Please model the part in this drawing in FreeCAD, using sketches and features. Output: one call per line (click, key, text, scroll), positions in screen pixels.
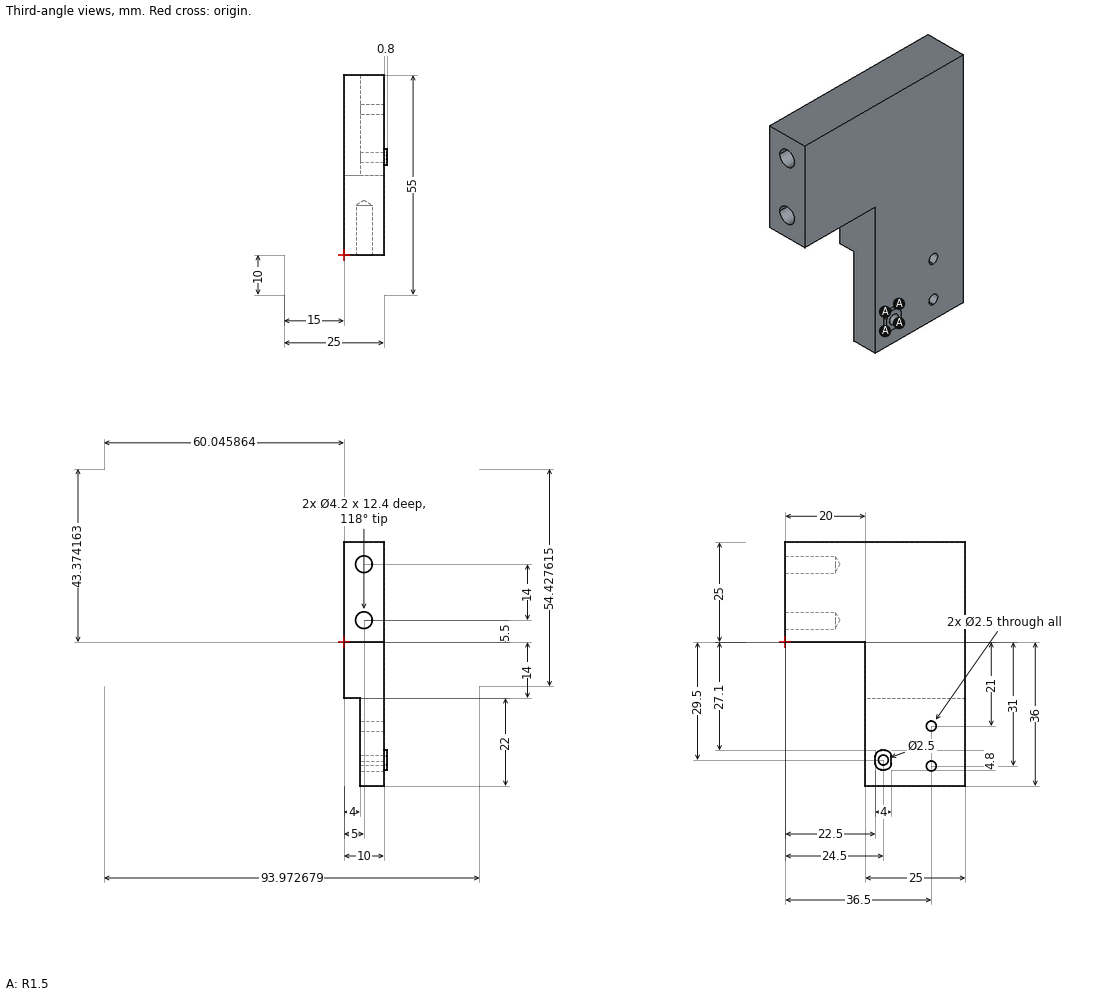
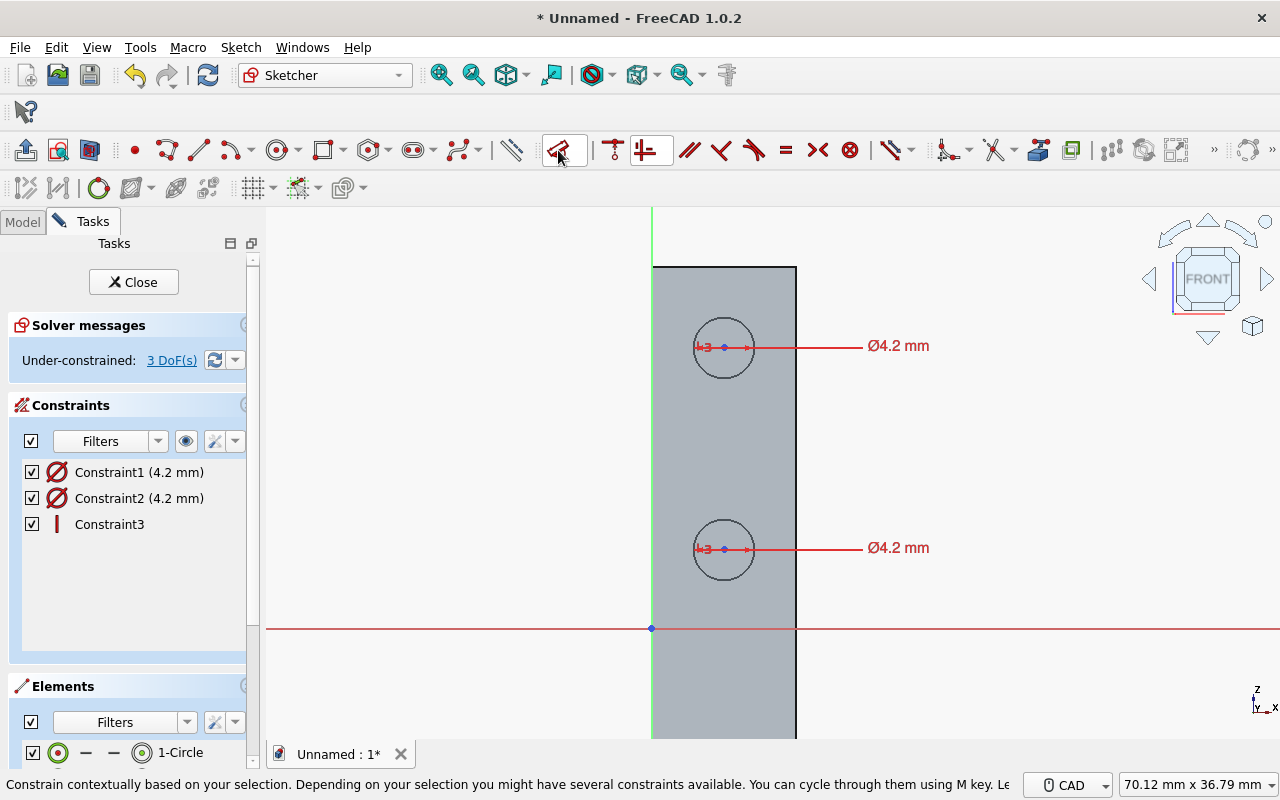
click(724, 550)
click(688, 663)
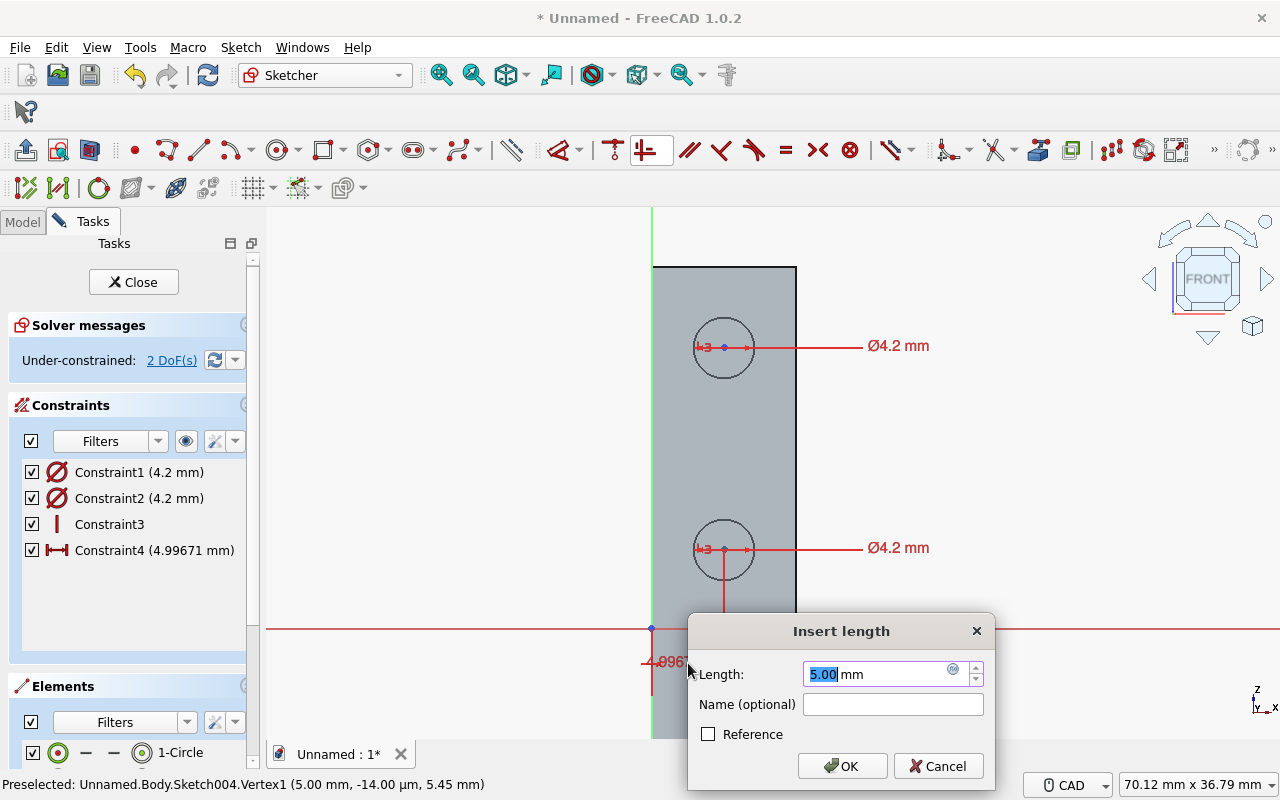
text(5)
key(Return)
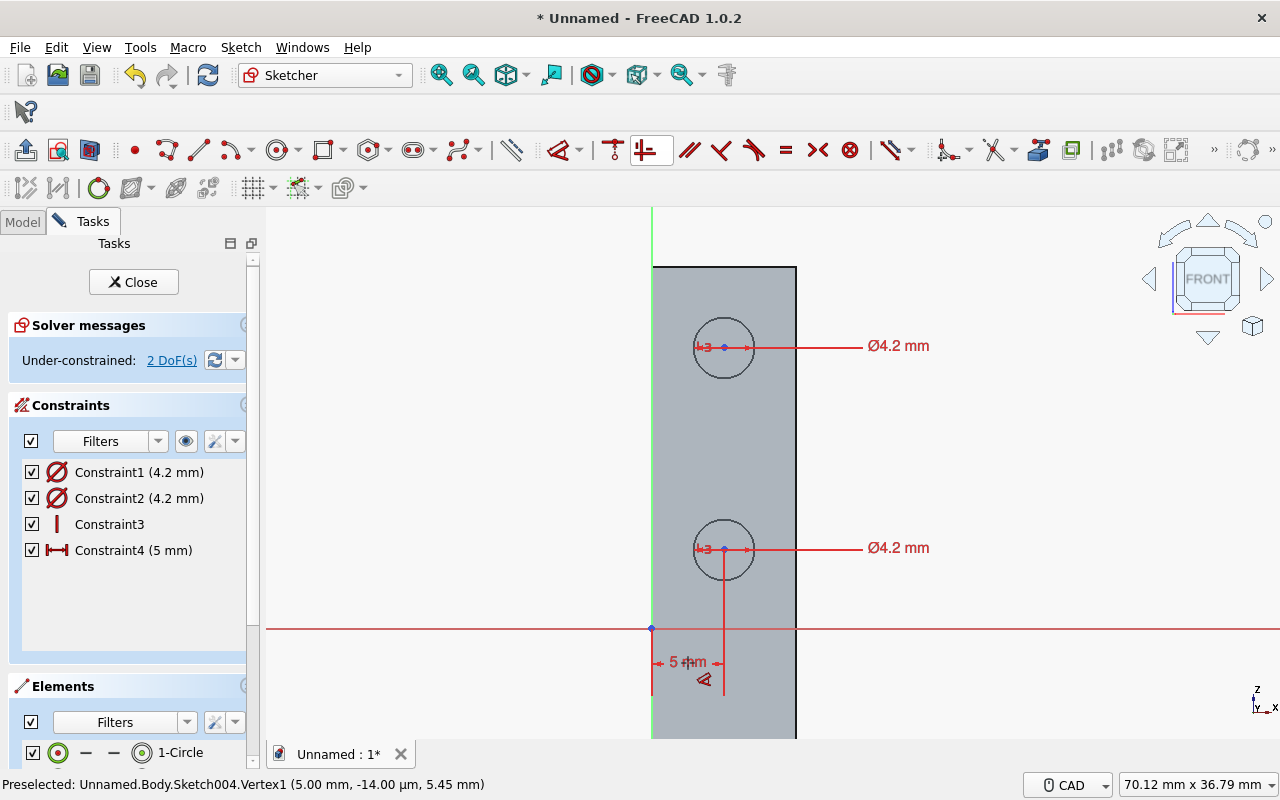
click(724, 550)
click(618, 589)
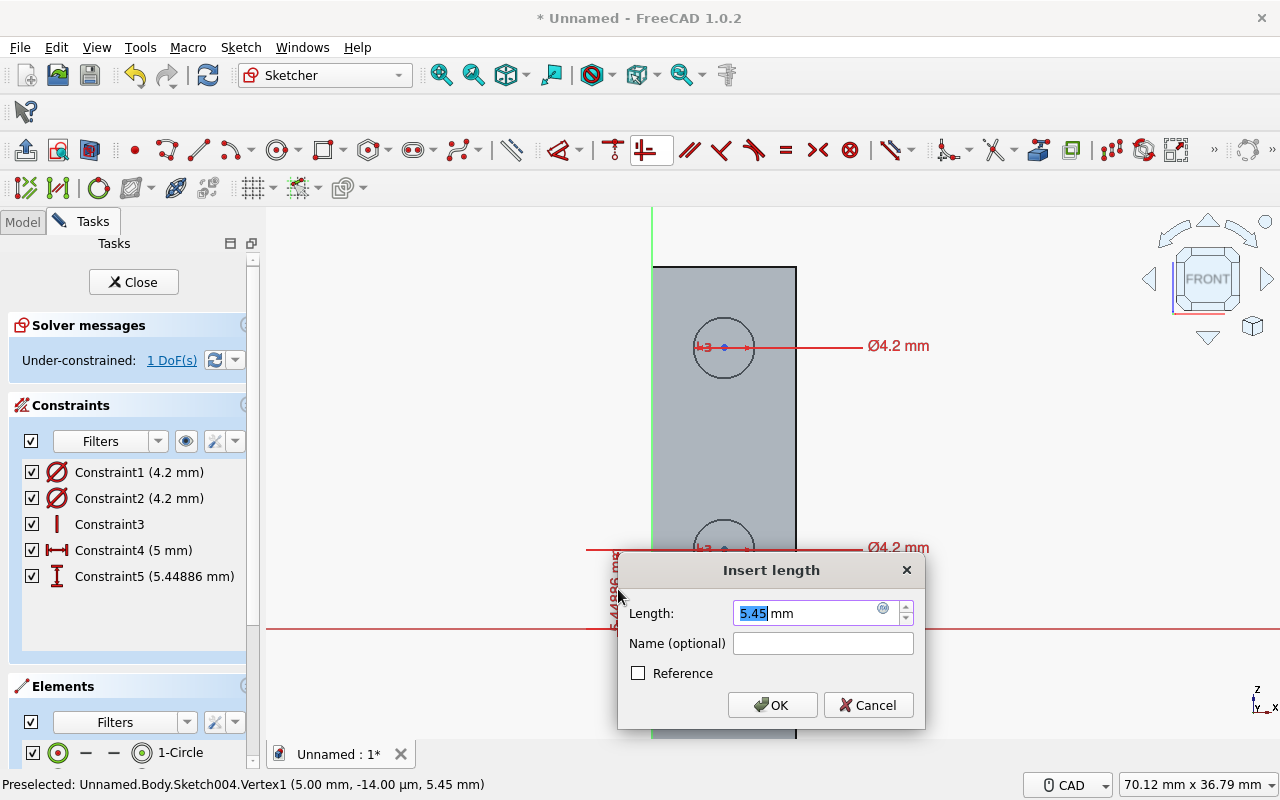
text(5.5)
key(Return)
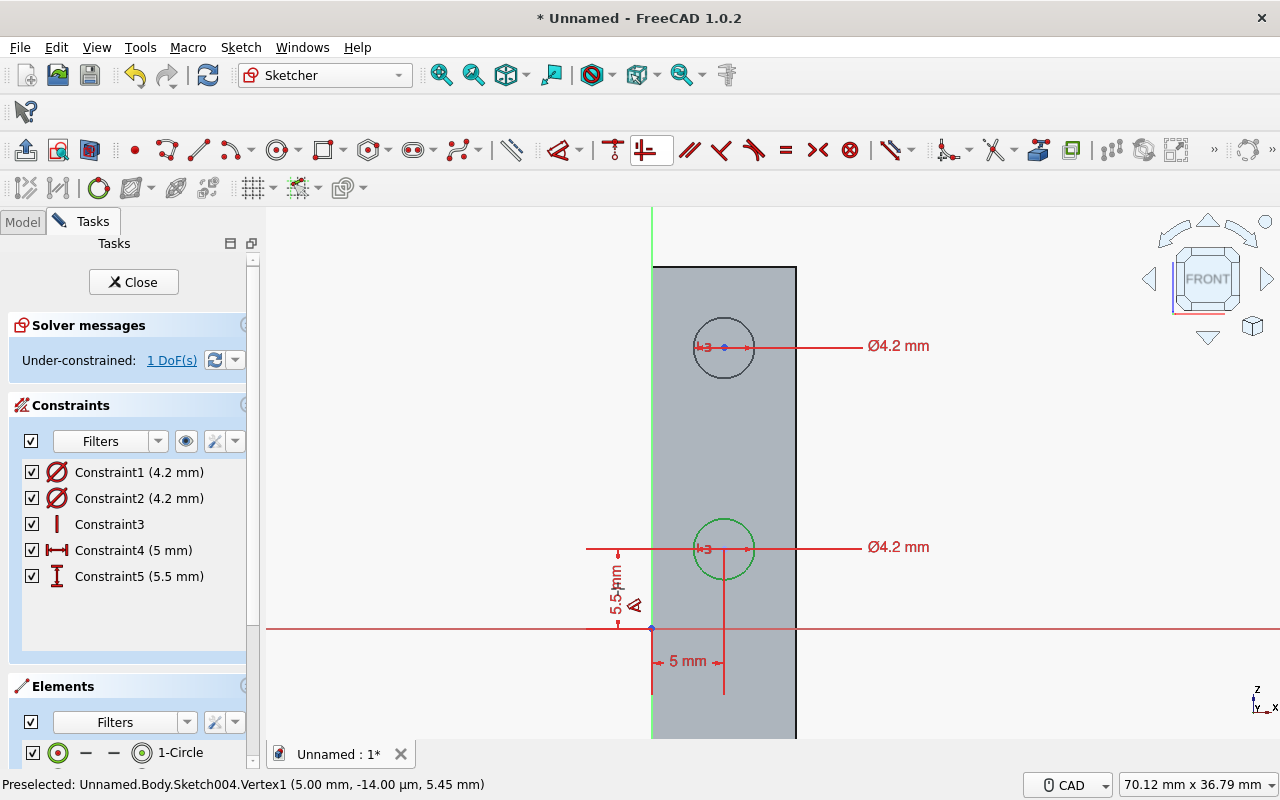
click(724, 549)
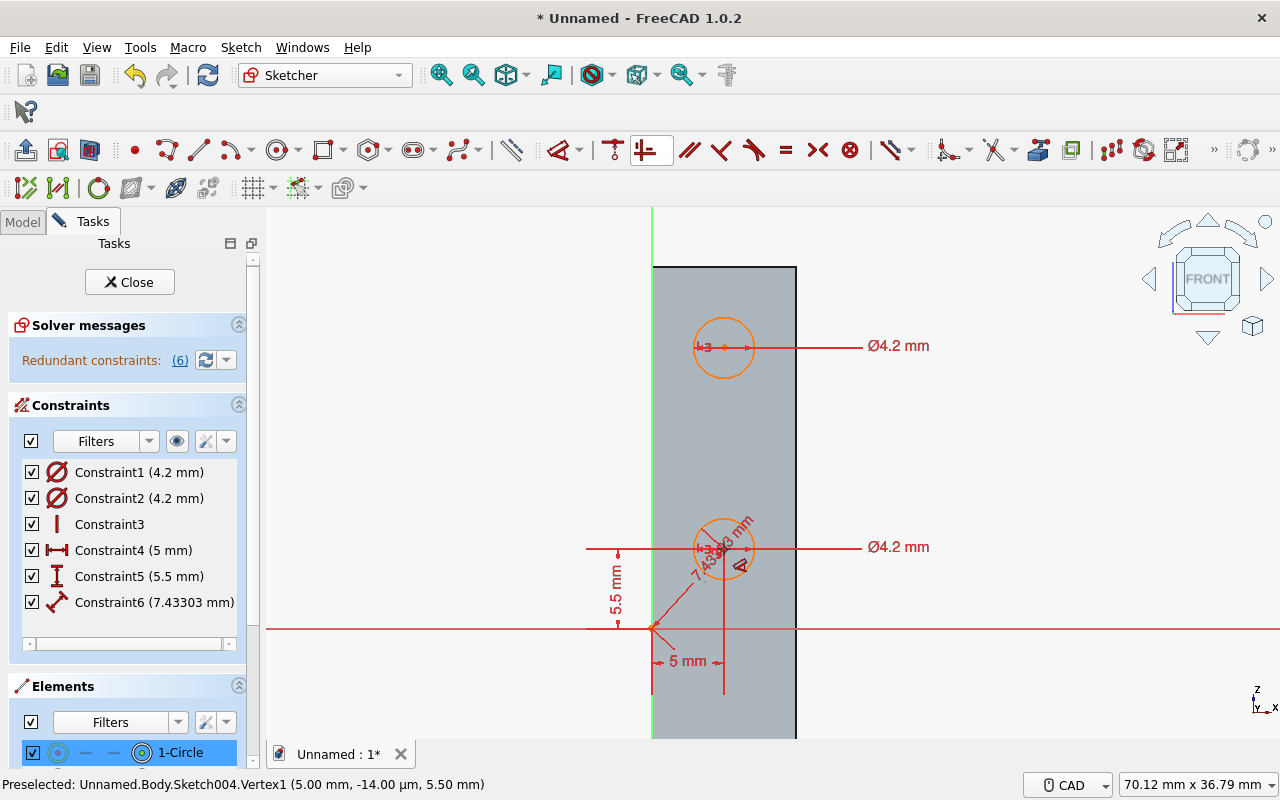
click(724, 348)
click(758, 449)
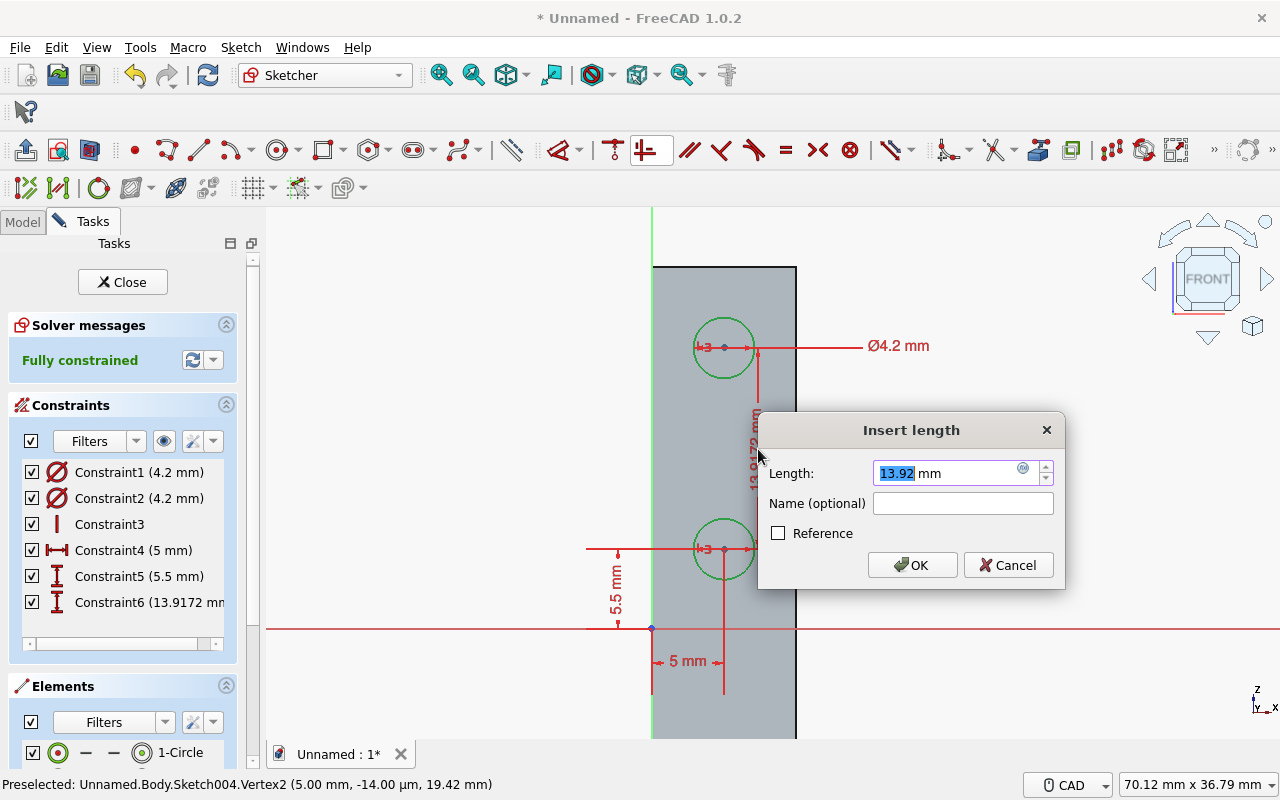
text(14)
key(Return)
key(Escape)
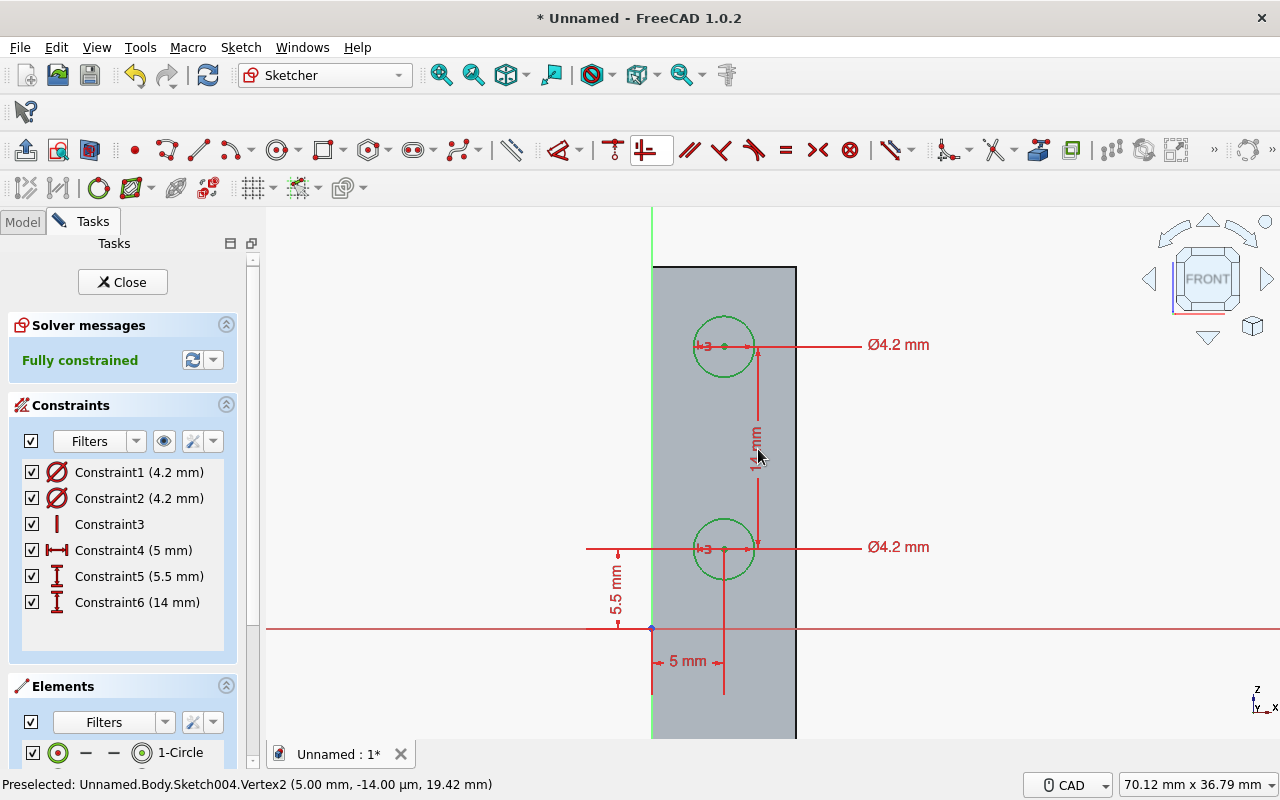
click(123, 282)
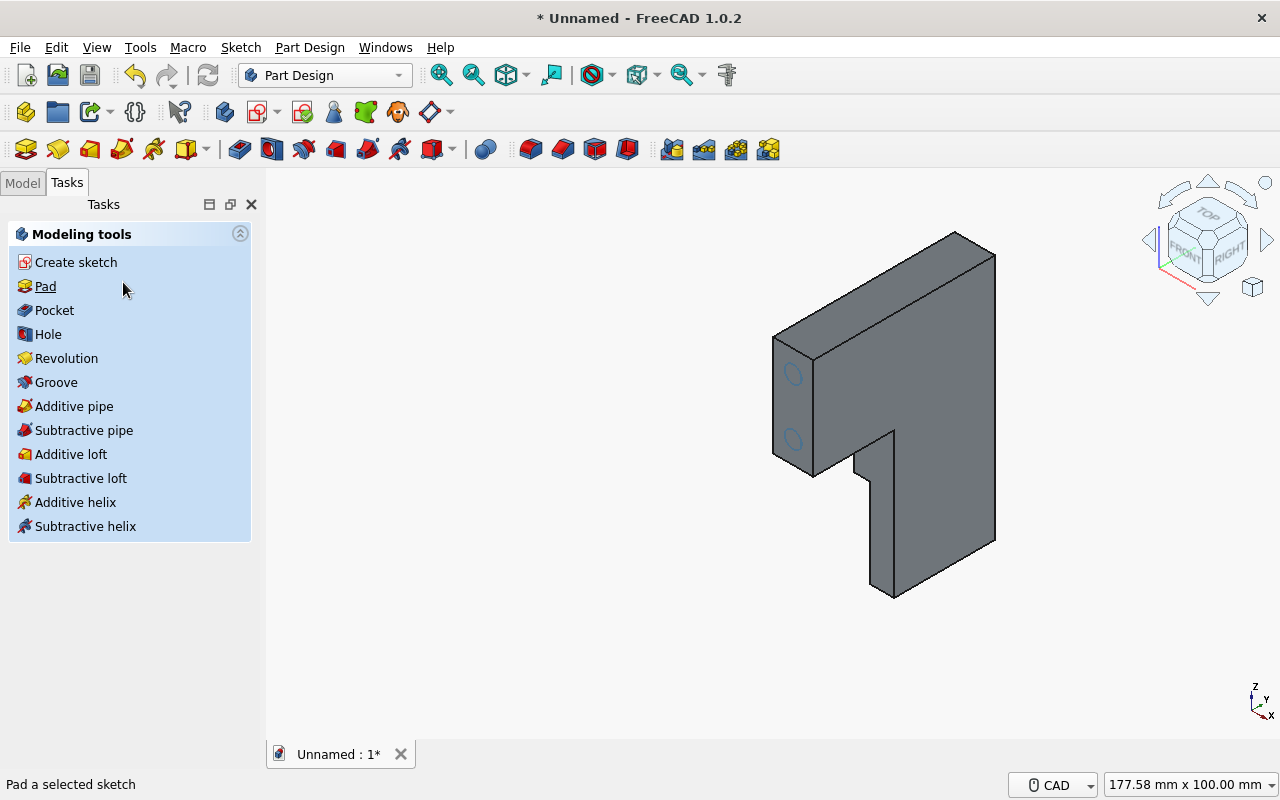
click(272, 150)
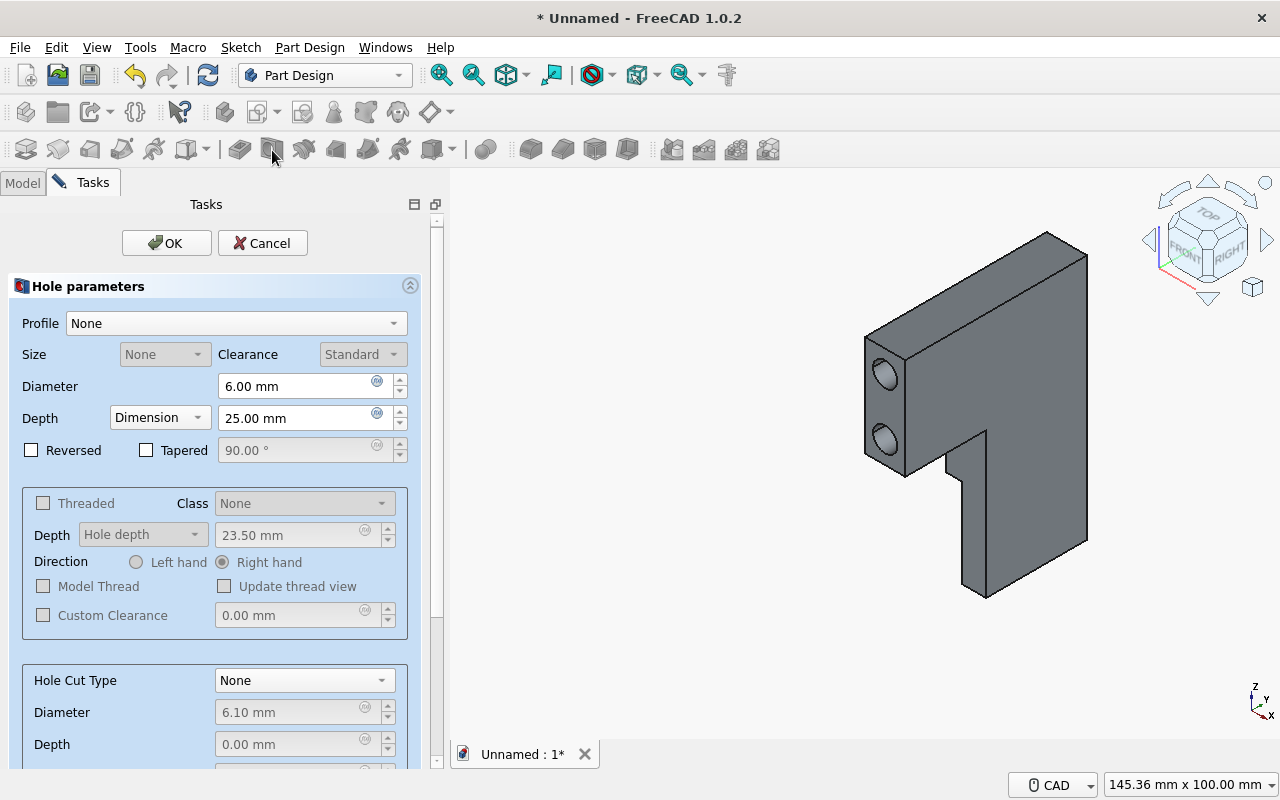
triple_click(305, 386)